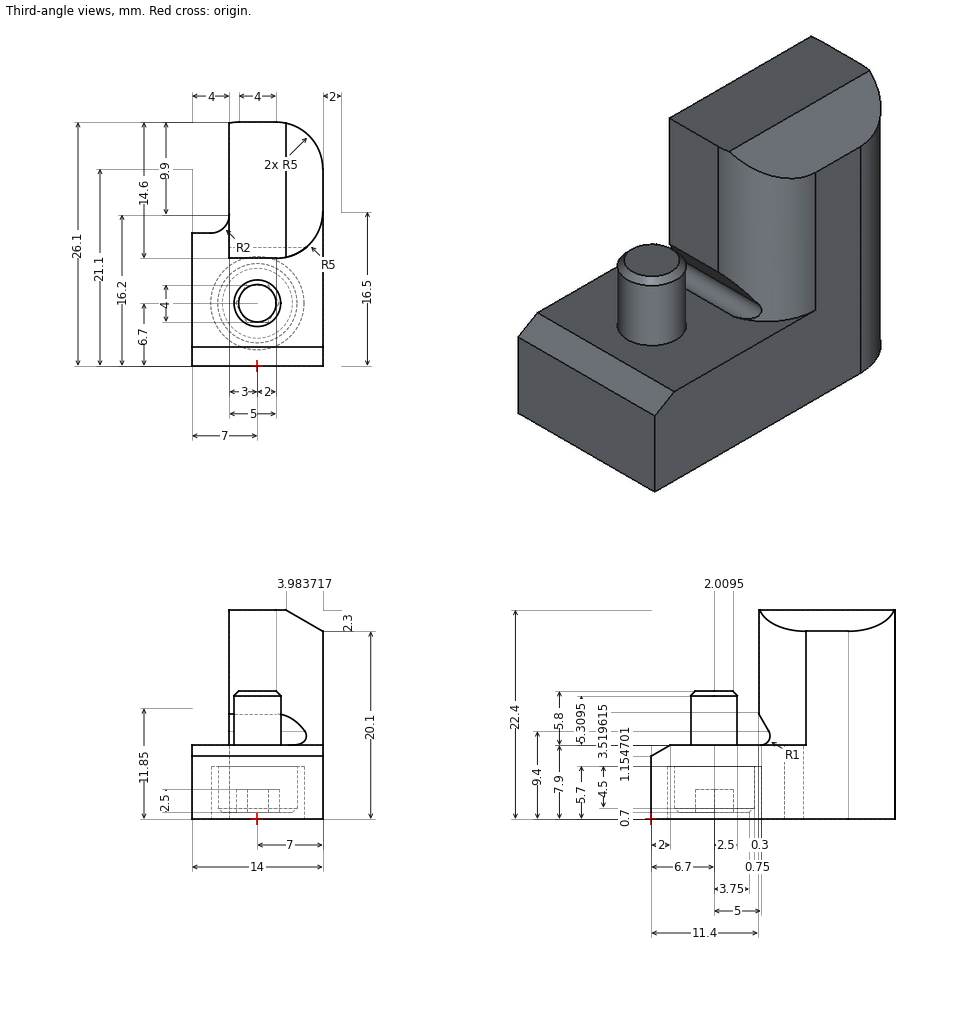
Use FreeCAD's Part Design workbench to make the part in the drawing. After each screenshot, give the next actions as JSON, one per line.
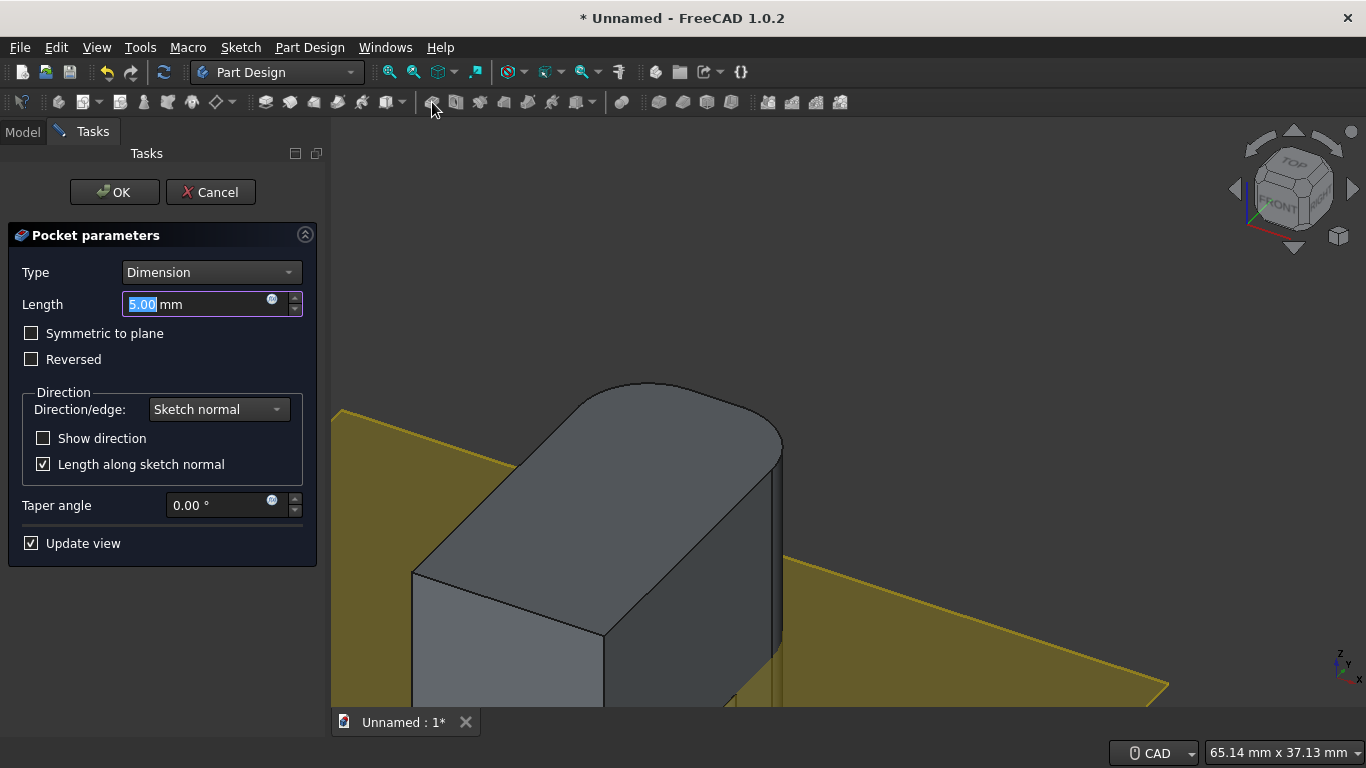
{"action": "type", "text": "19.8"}
{"action": "key", "text": "Tab"}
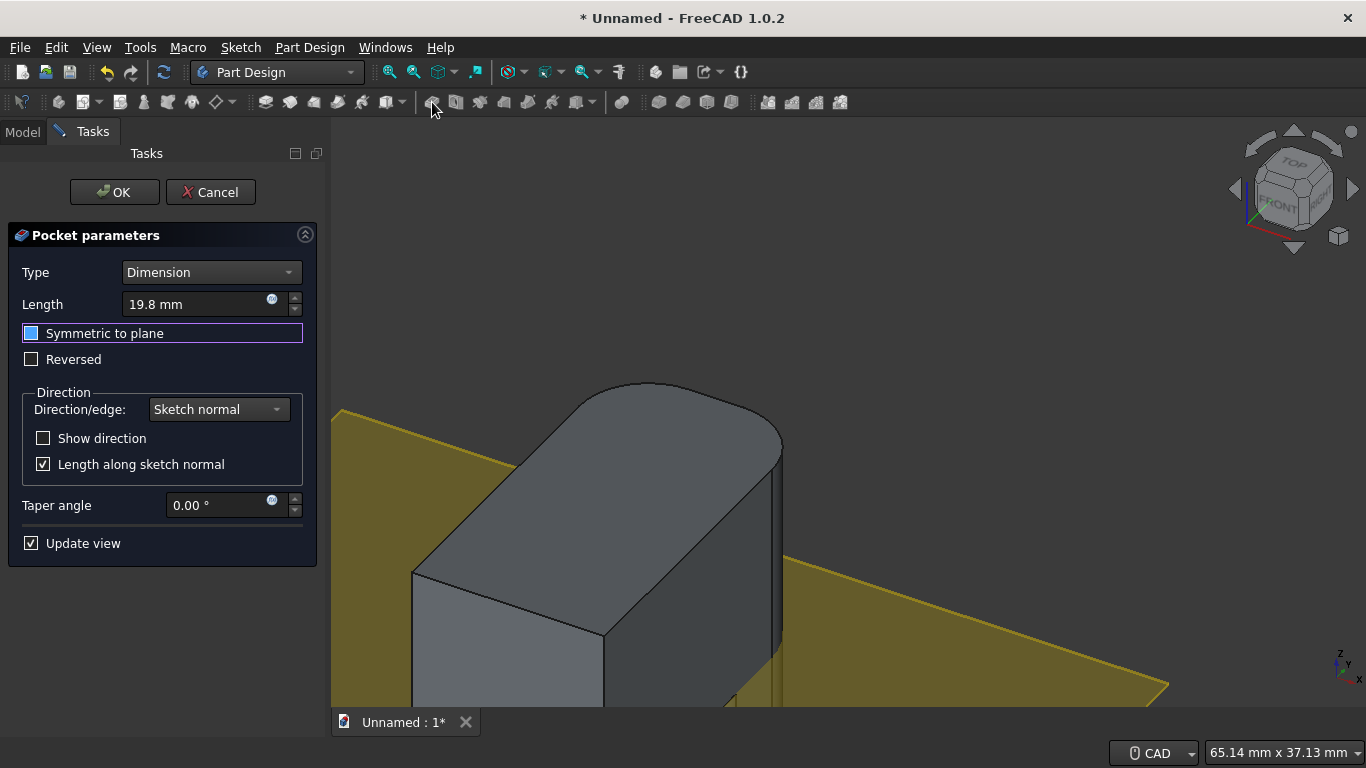
{"action": "left_click", "coordinate": [30, 359]}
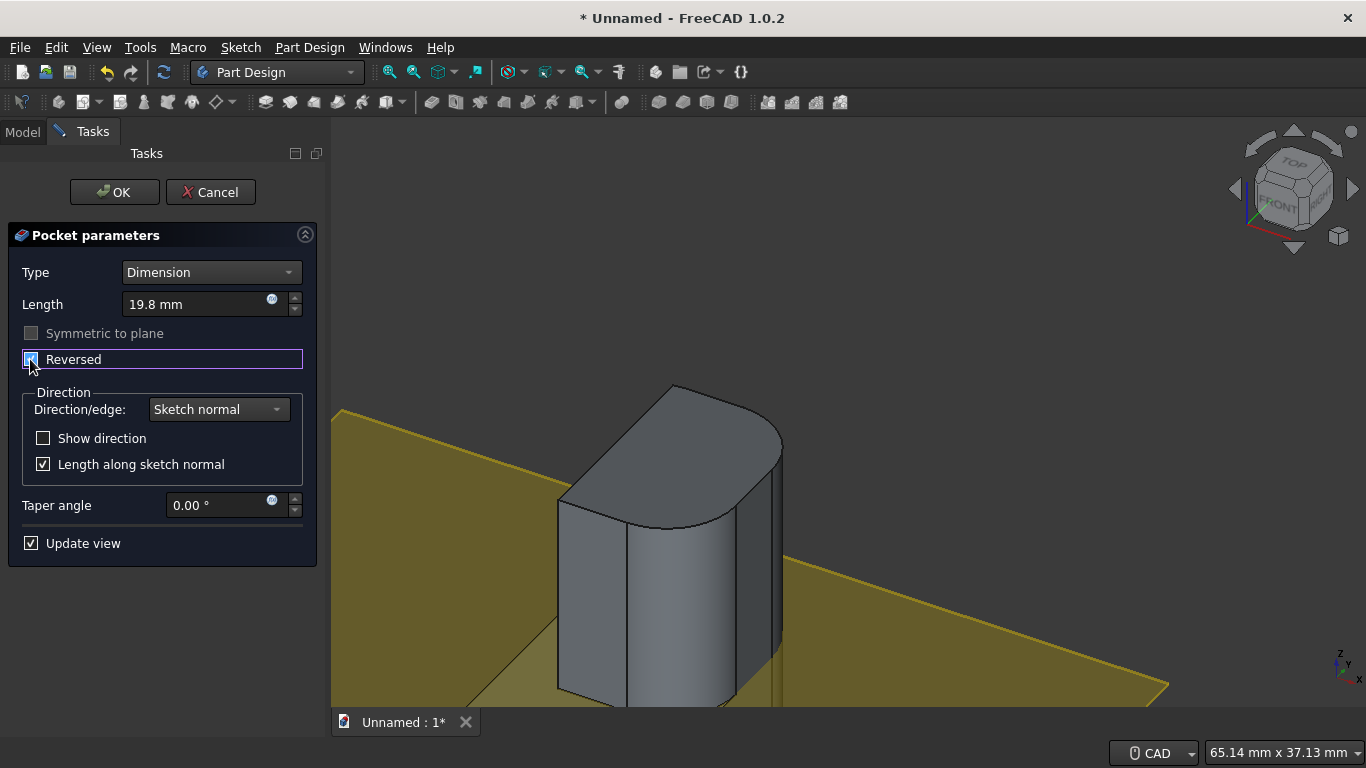
{"action": "left_click", "coordinate": [115, 192]}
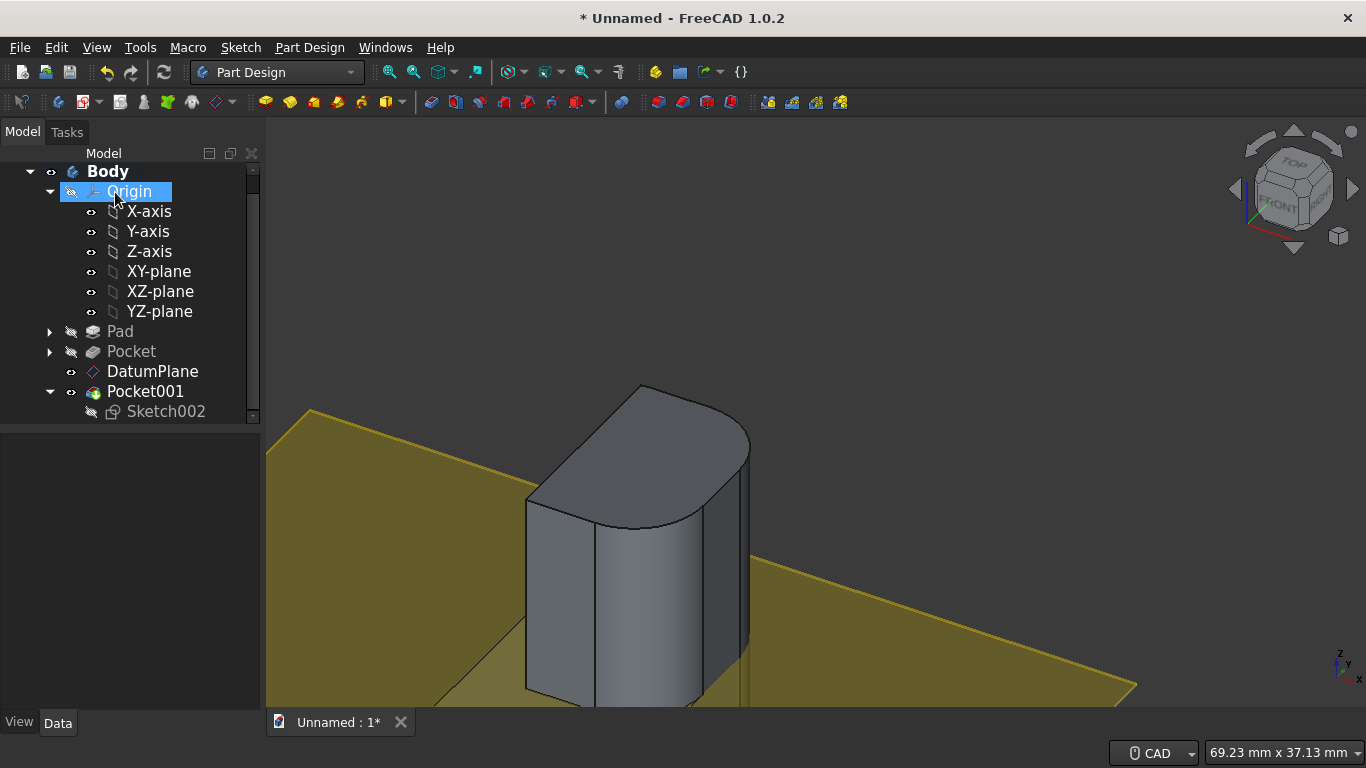
{"action": "left_click", "coordinate": [116, 372]}
{"action": "key", "text": "space"}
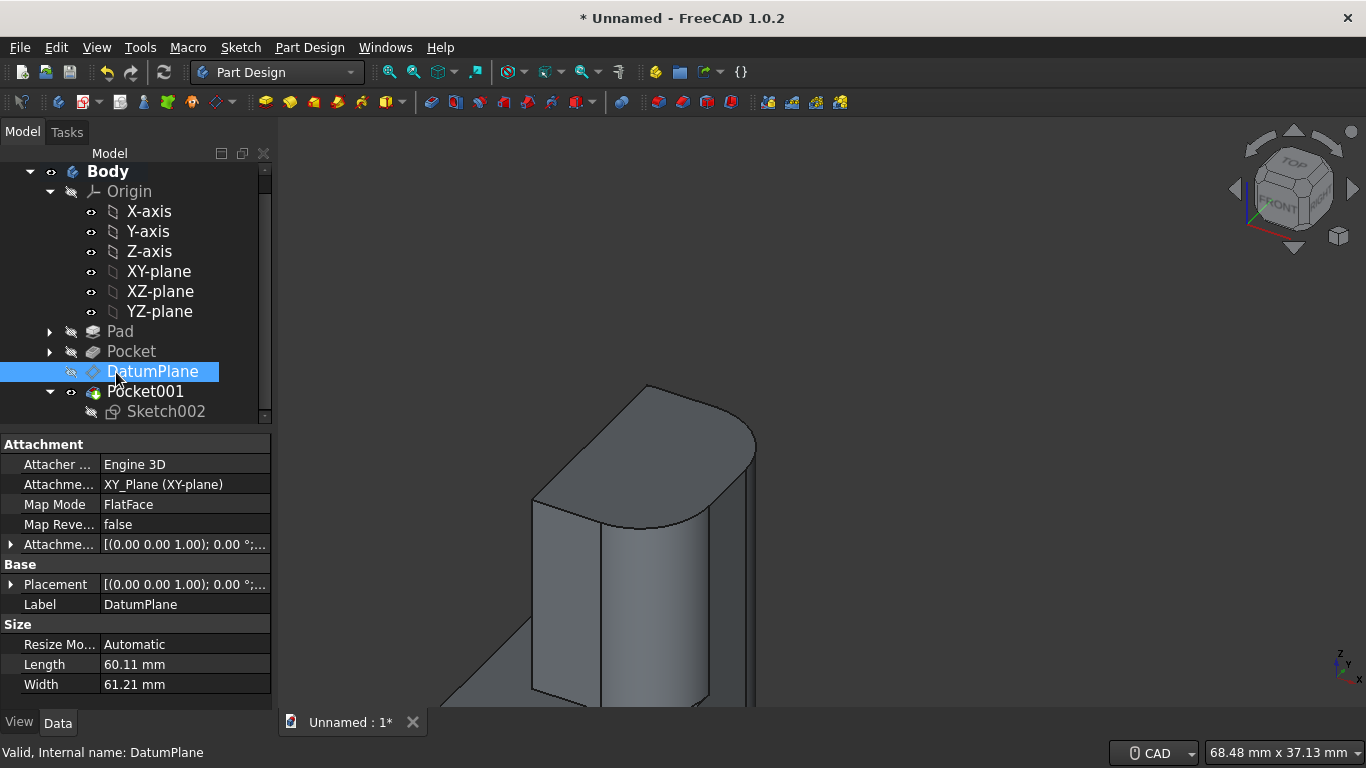
{"action": "left_click", "coordinate": [390, 72]}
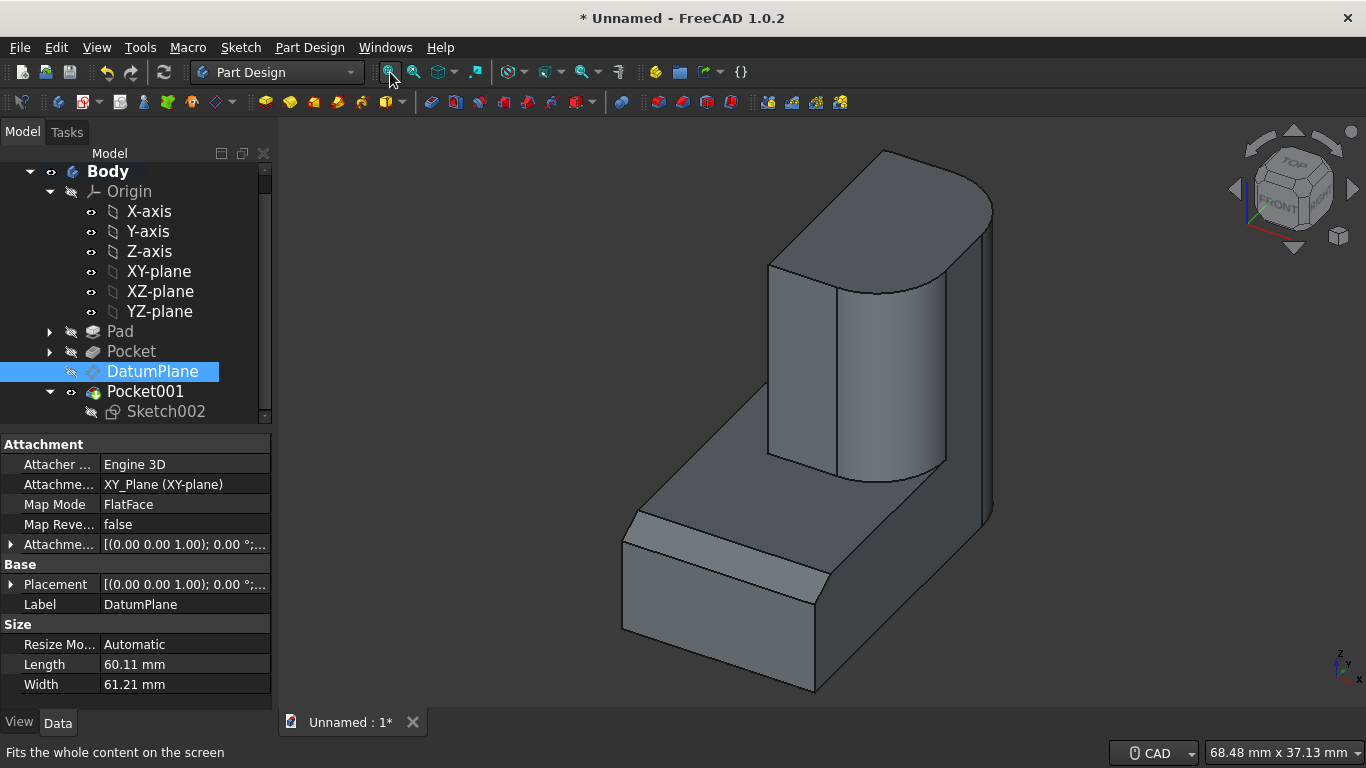
{"action": "left_click", "coordinate": [318, 667]}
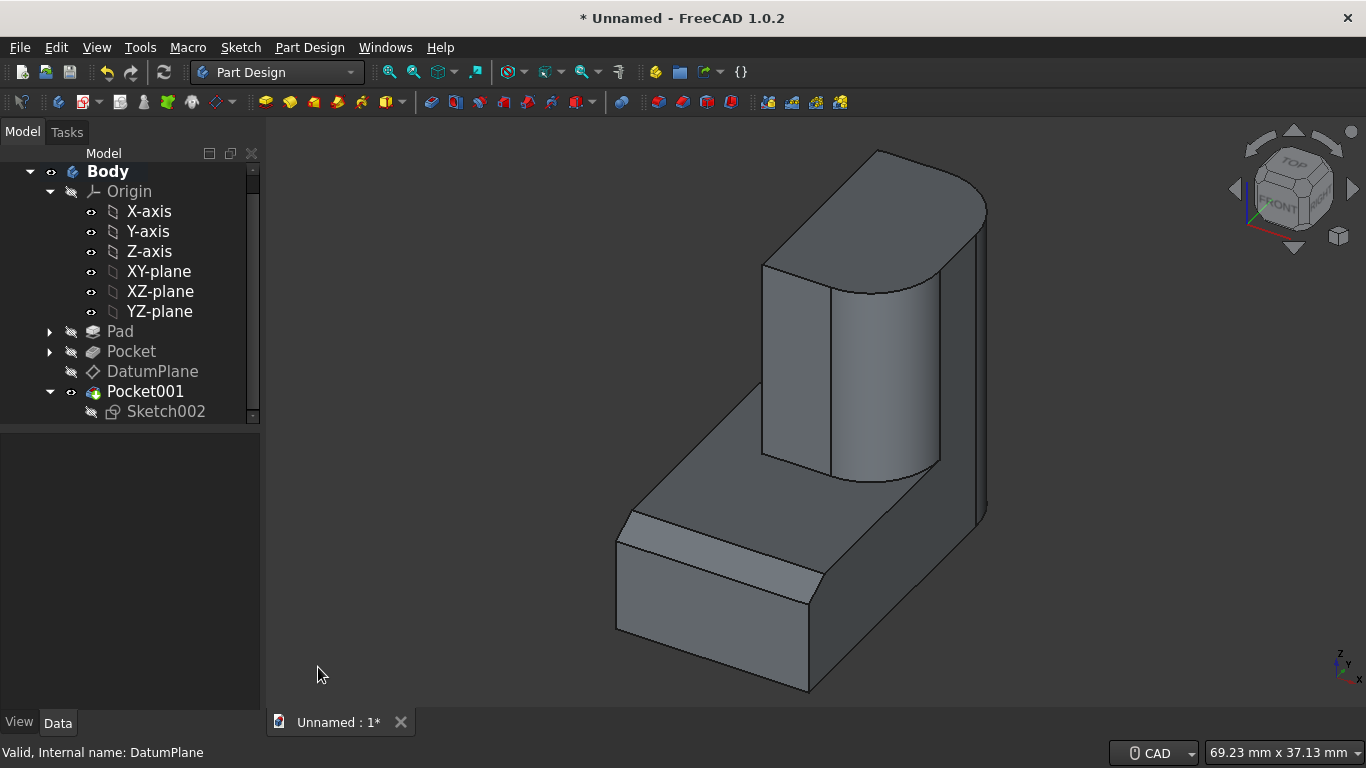
{"action": "left_click", "coordinate": [84, 102]}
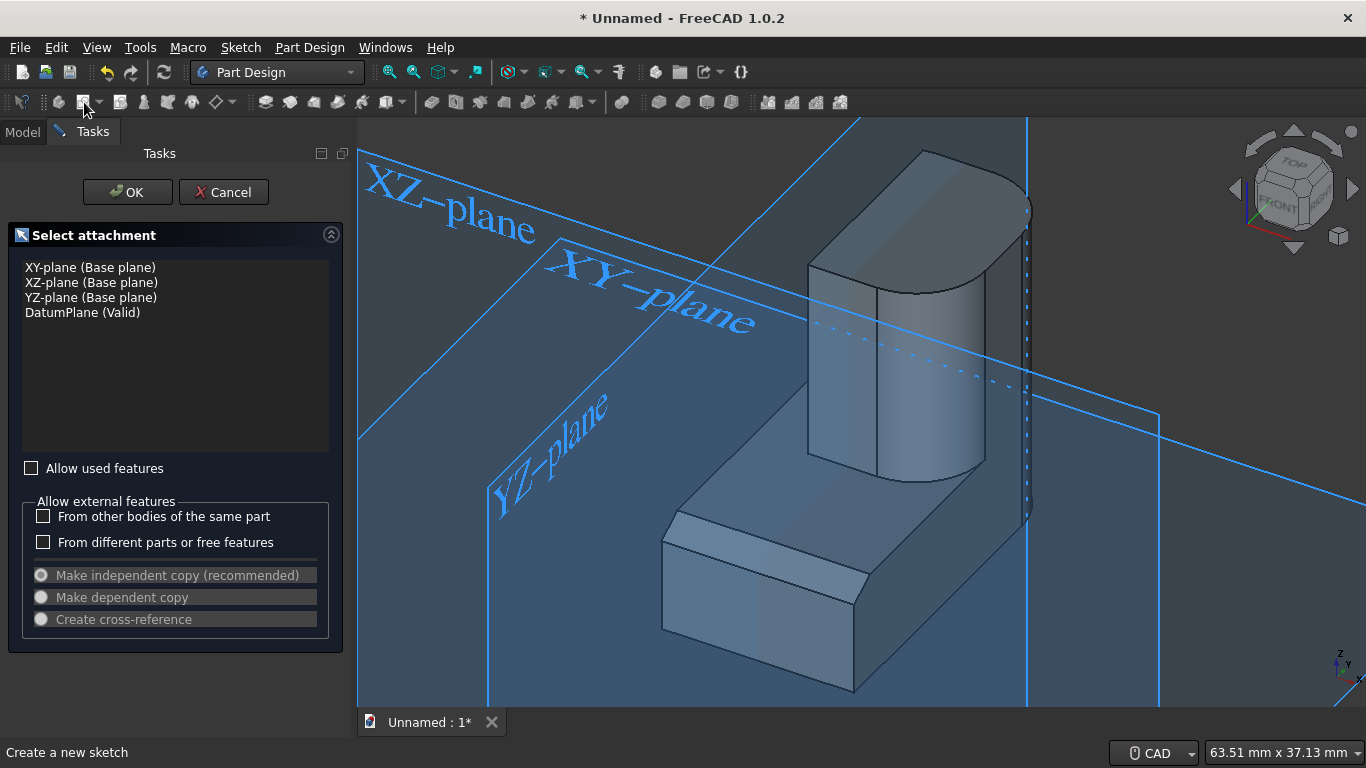
{"action": "left_click", "coordinate": [82, 298]}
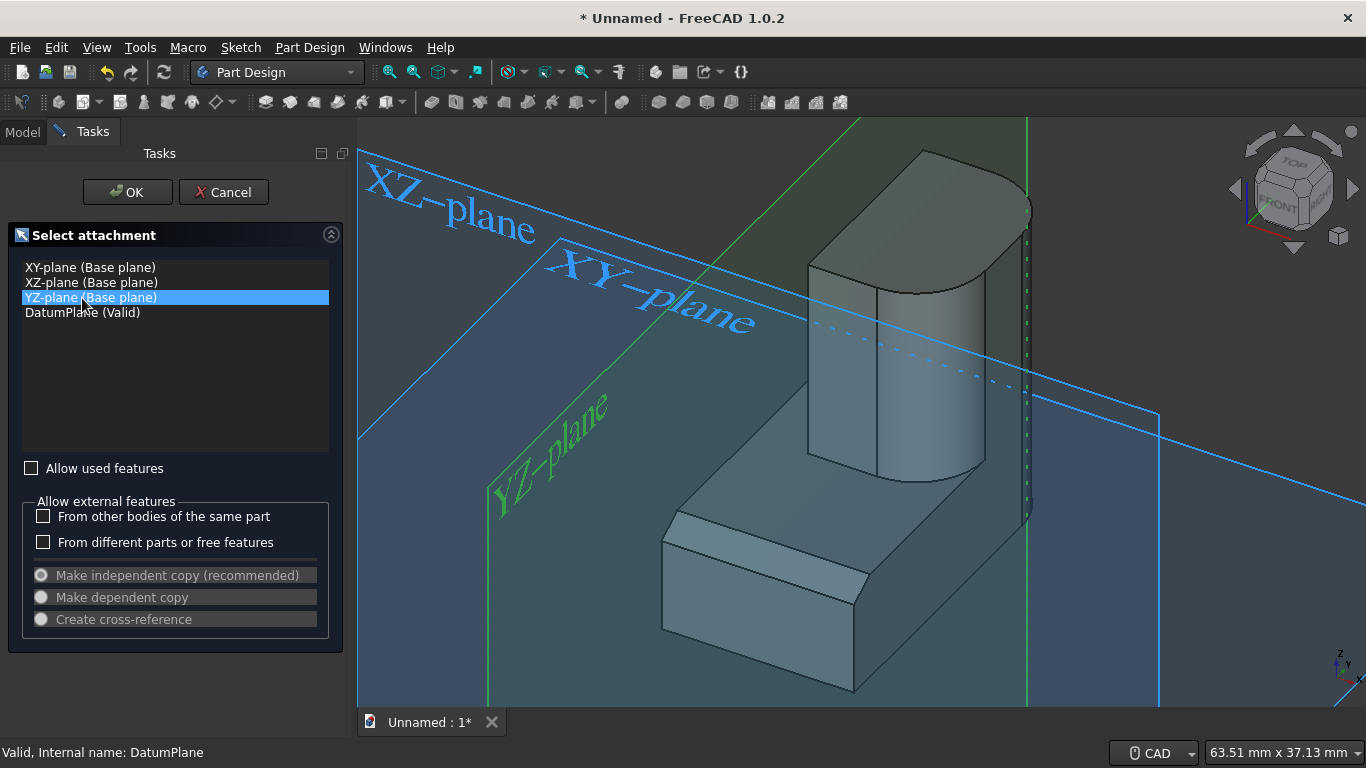
{"action": "left_click", "coordinate": [128, 192]}